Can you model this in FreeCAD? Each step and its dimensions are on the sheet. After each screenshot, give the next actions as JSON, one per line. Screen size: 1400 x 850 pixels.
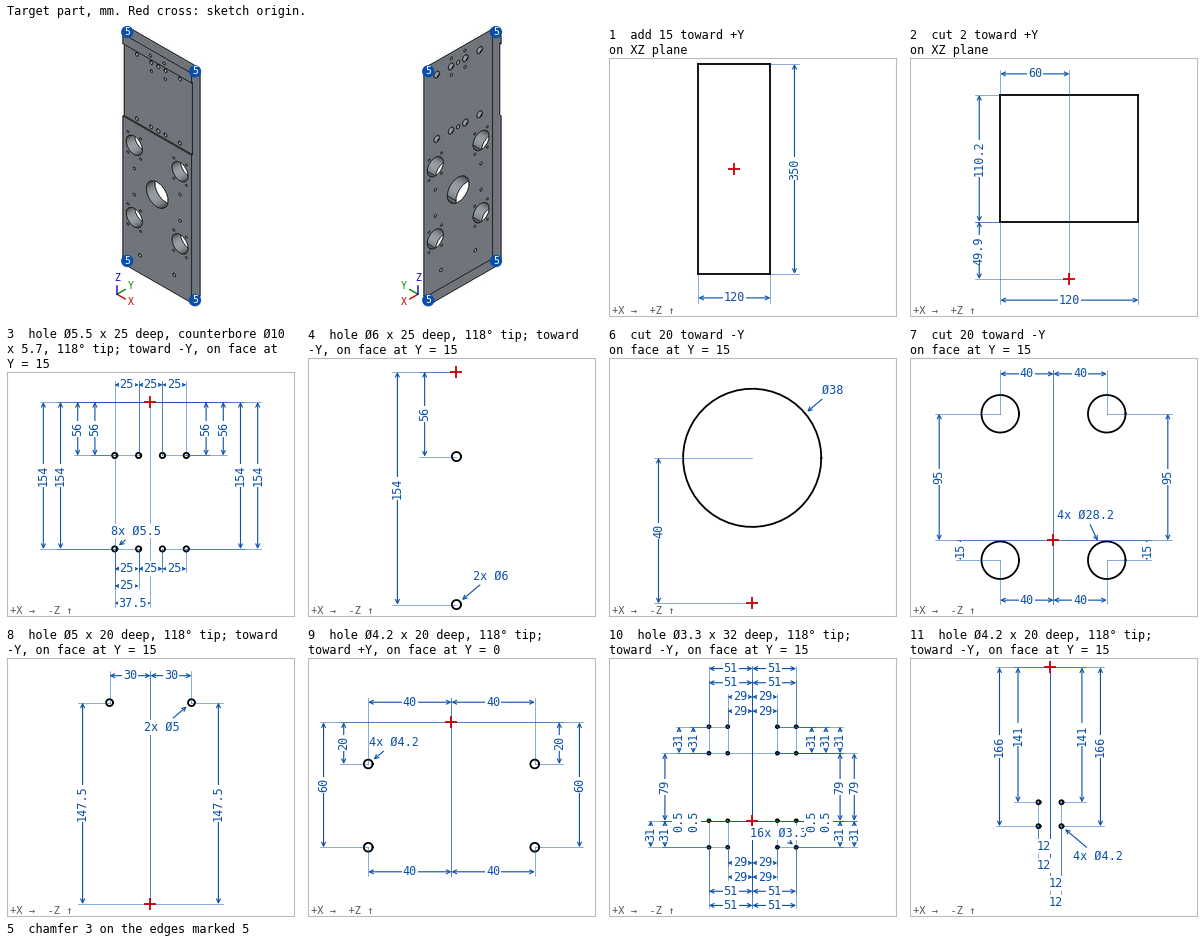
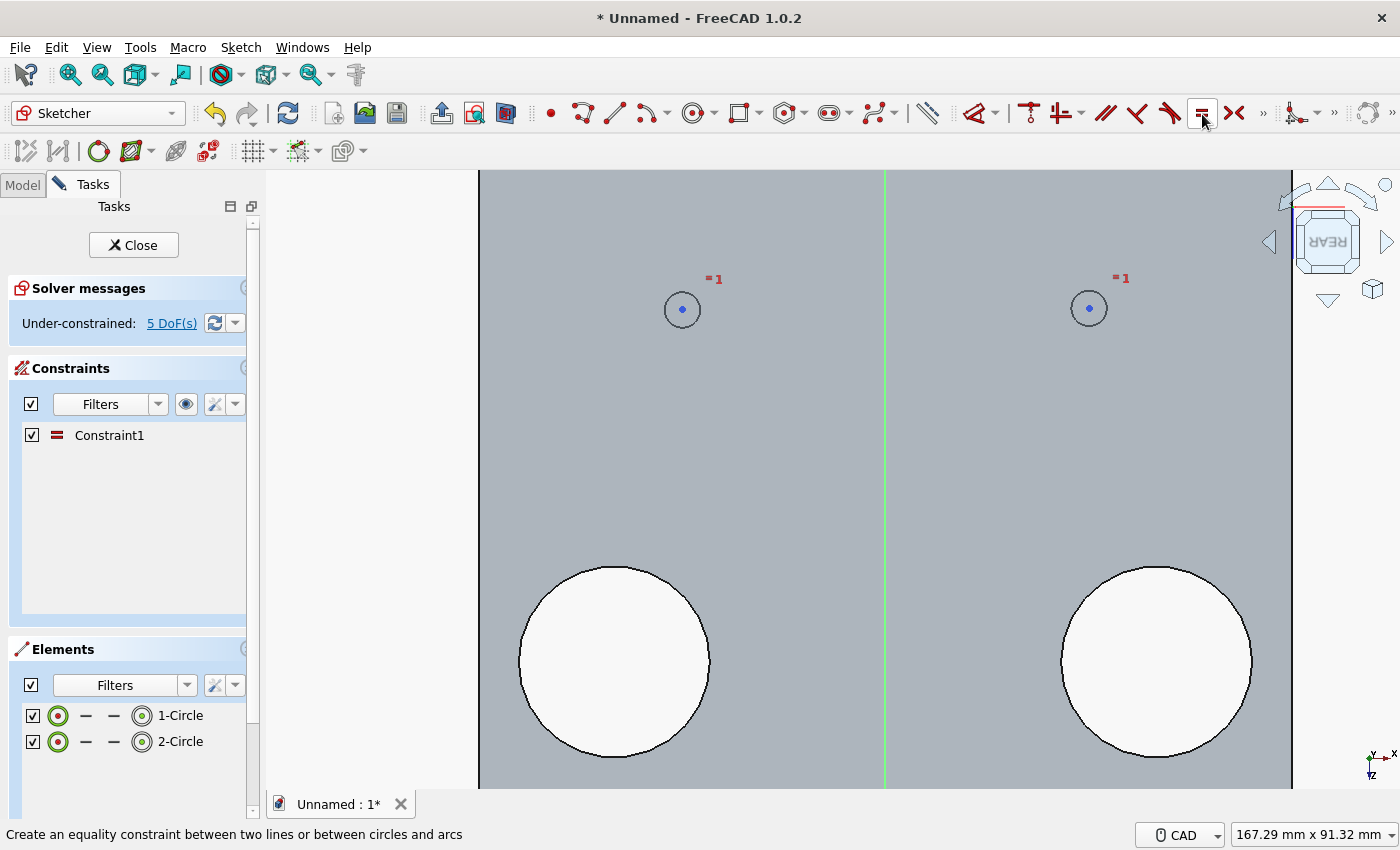
{"action": "left_click", "coordinate": [974, 114]}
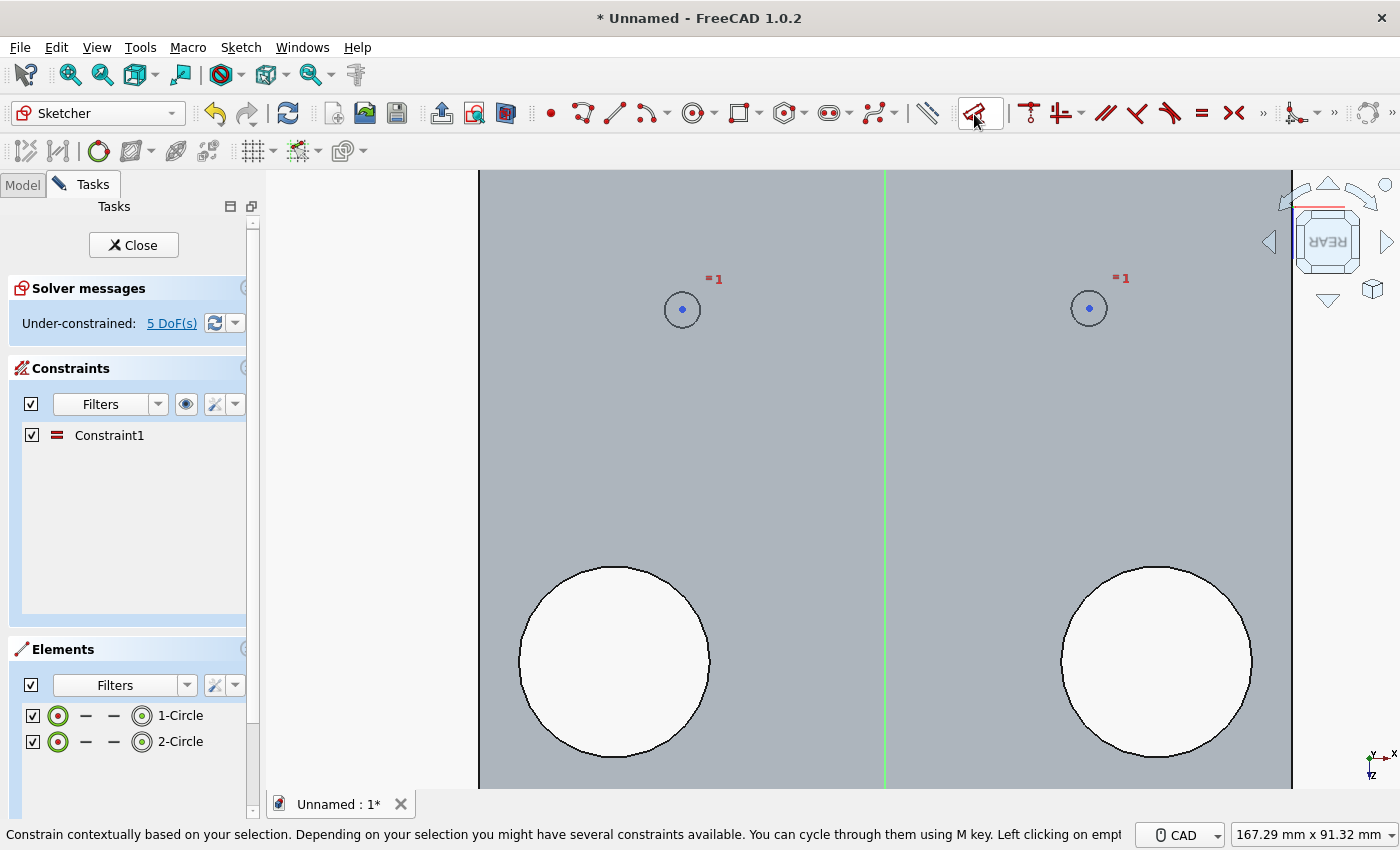
{"action": "left_click", "coordinate": [1102, 296]}
{"action": "left_click", "coordinate": [1125, 274]}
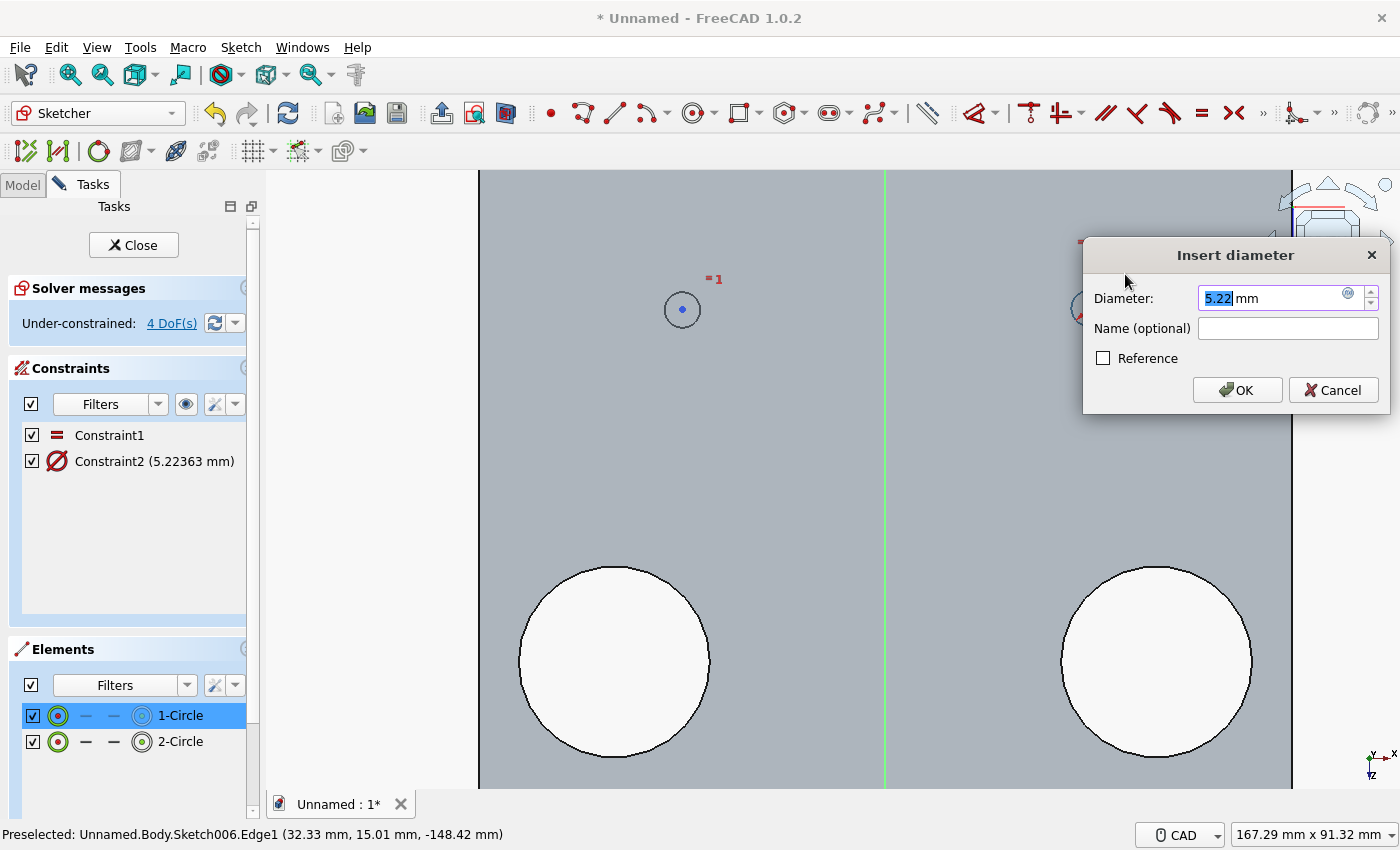
{"action": "type", "text": "5"}
{"action": "key", "text": "Return"}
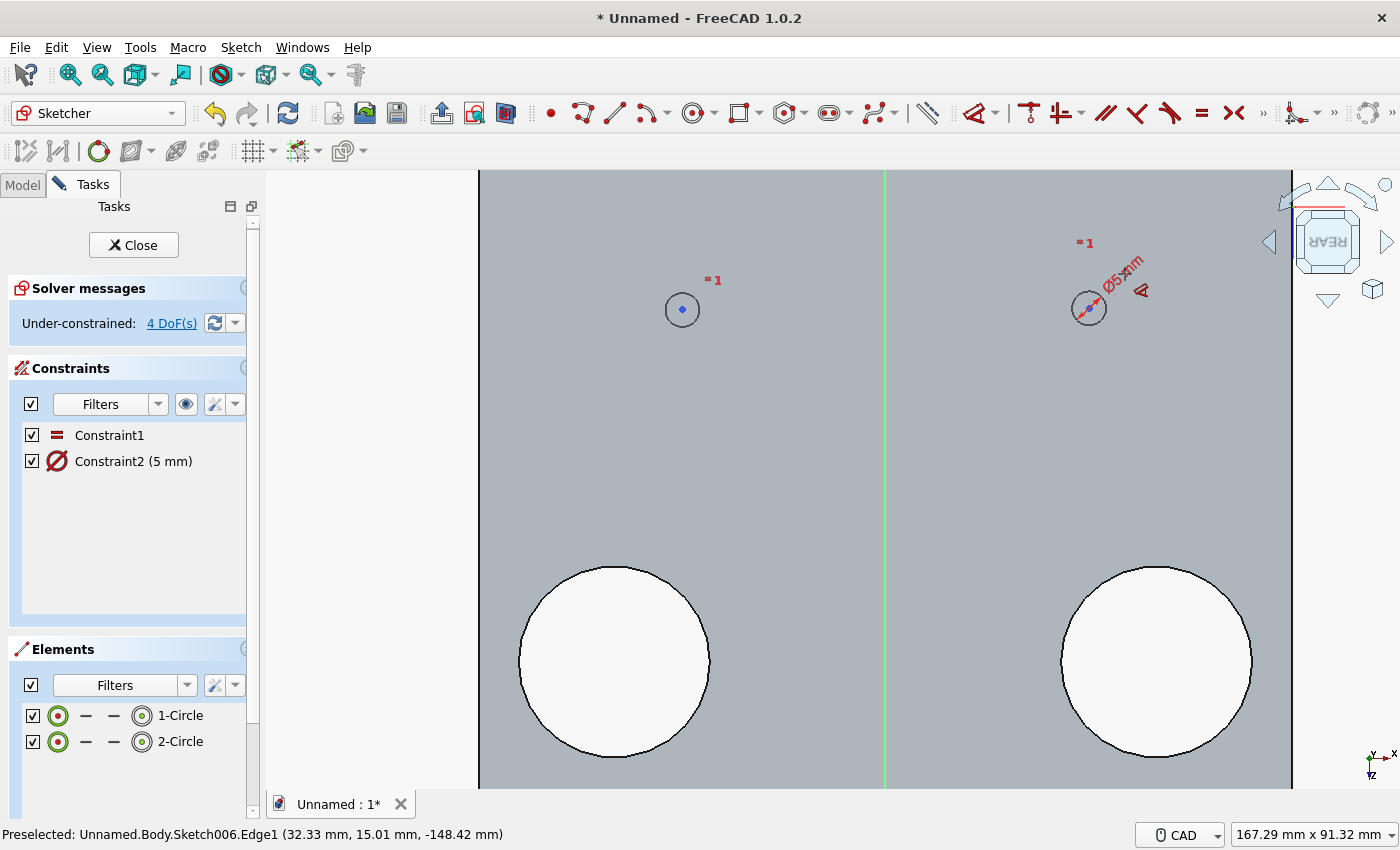
{"action": "left_click", "coordinate": [1089, 308]}
{"action": "left_click", "coordinate": [987, 274]}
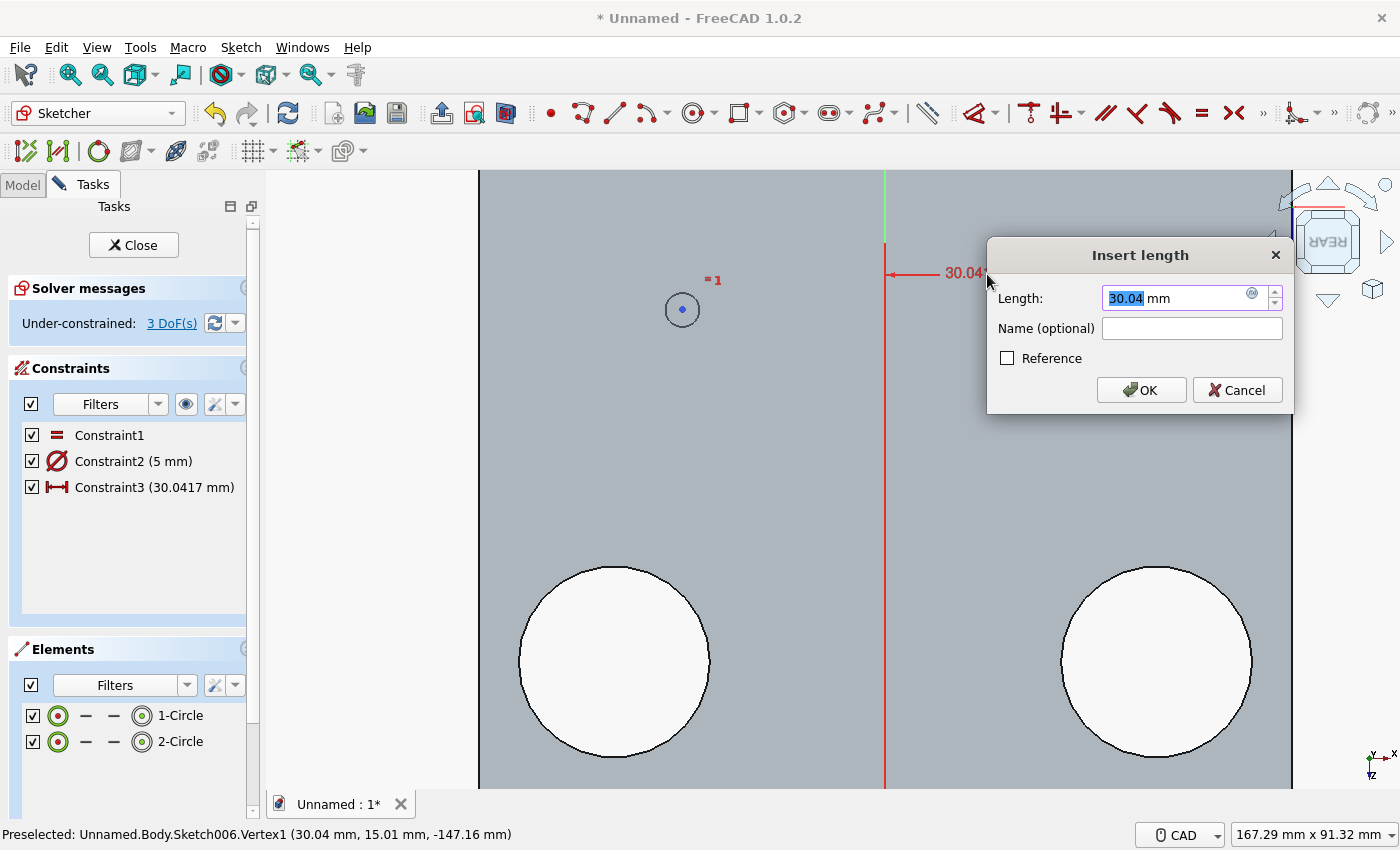
{"action": "type", "text": "30"}
{"action": "key", "text": "Return"}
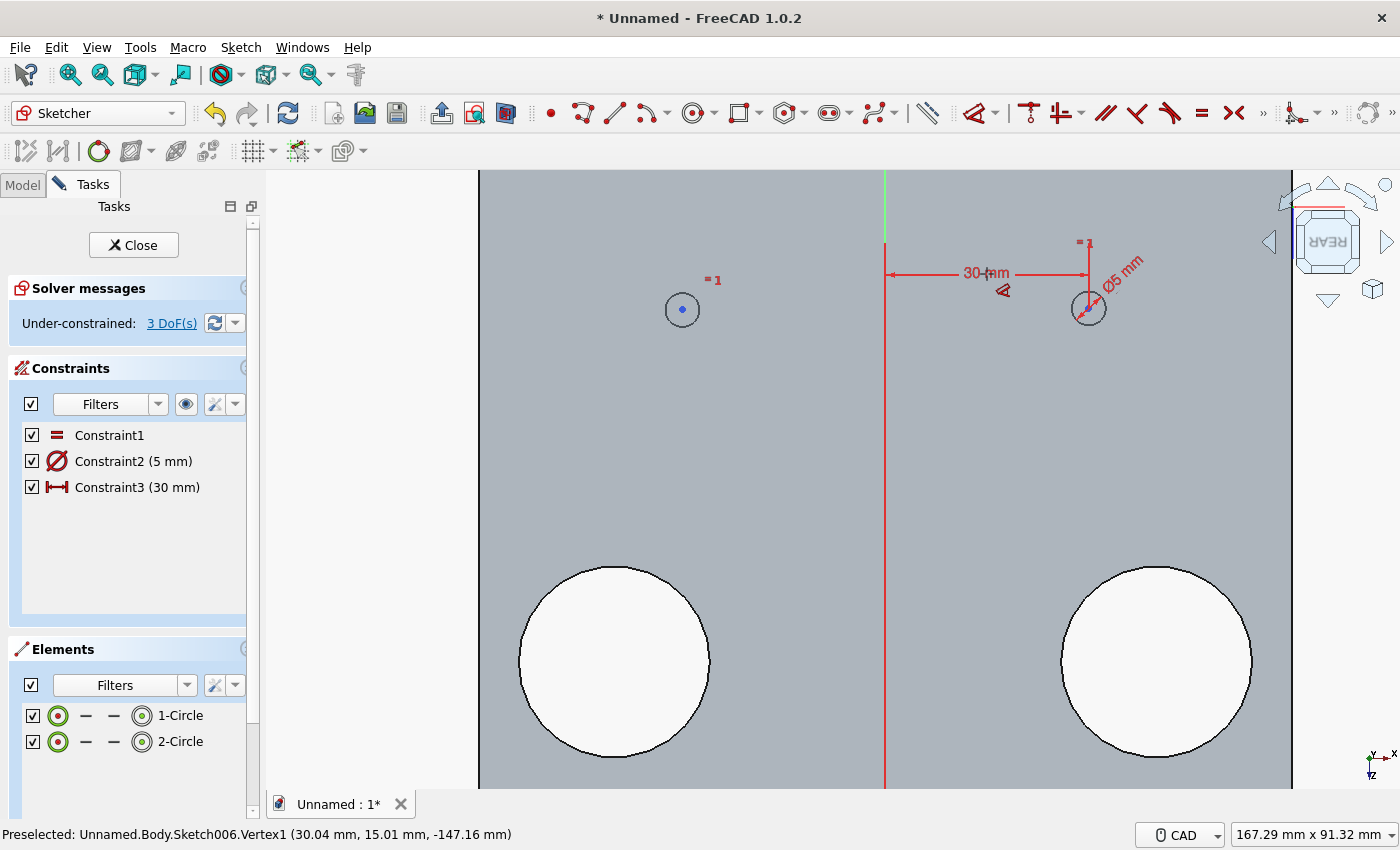
{"action": "left_click", "coordinate": [682, 310]}
{"action": "left_click", "coordinate": [784, 276]}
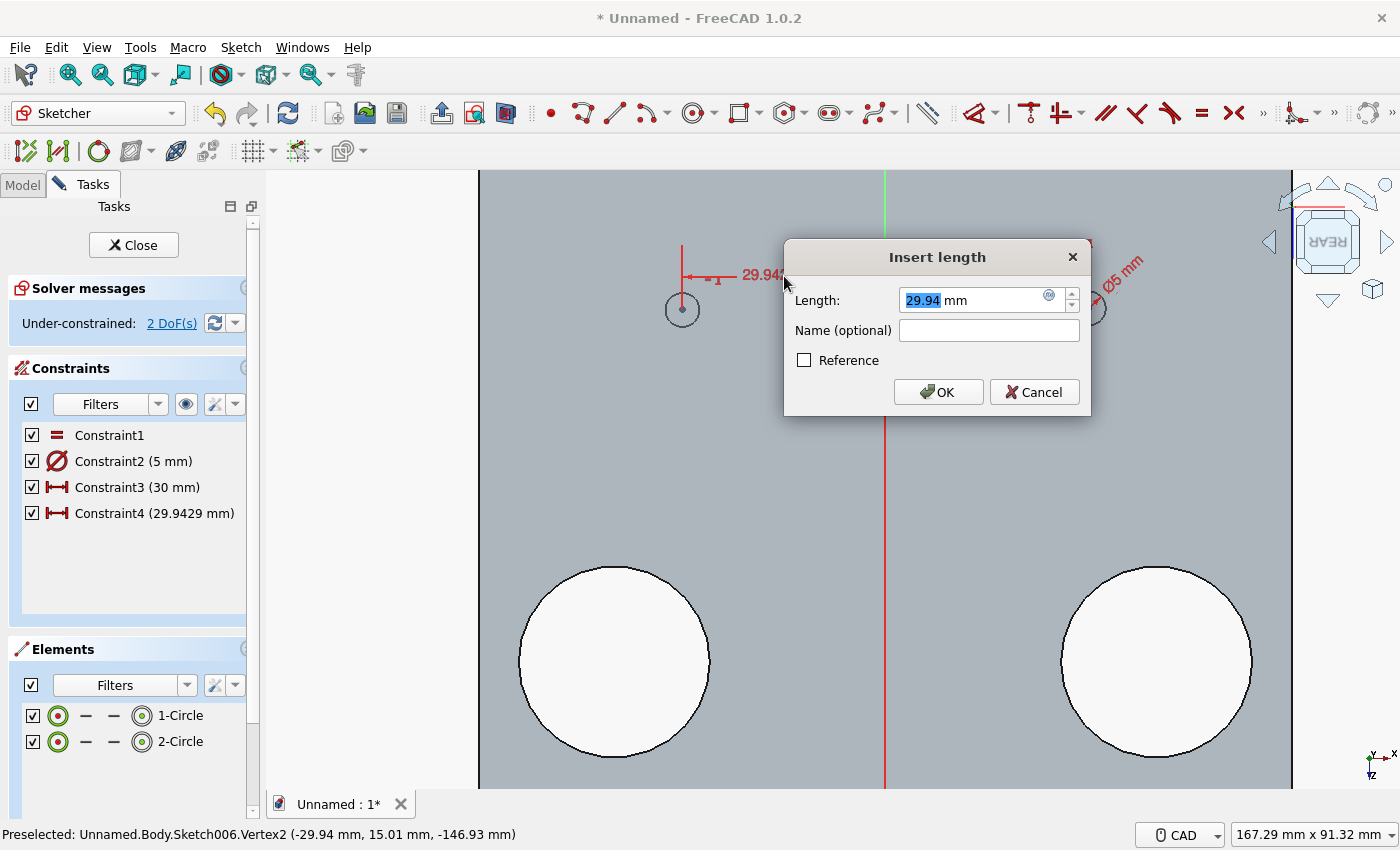
{"action": "type", "text": "30"}
{"action": "key", "text": "Return"}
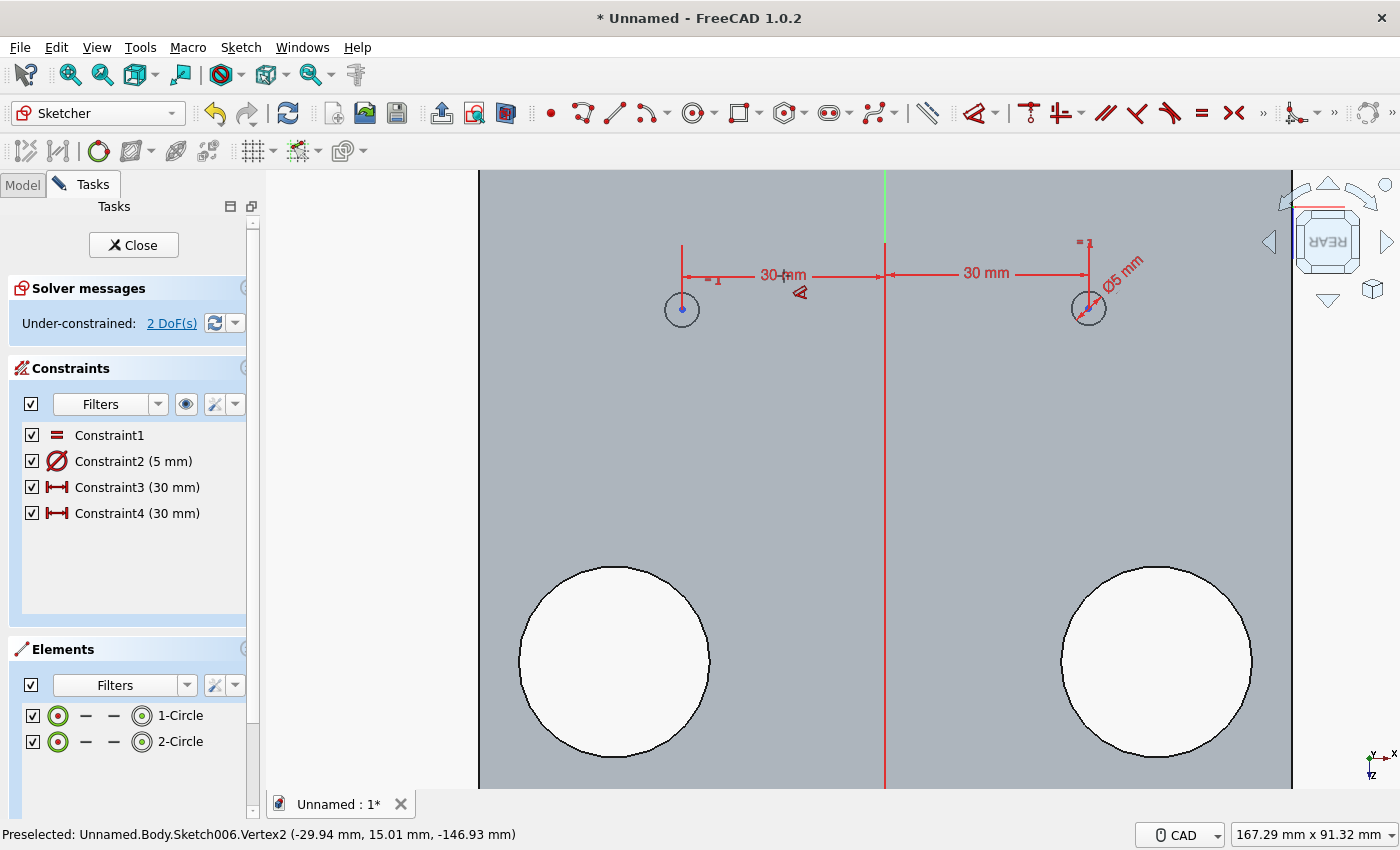
{"action": "left_click", "coordinate": [1089, 308]}
{"action": "left_click", "coordinate": [1123, 535]}